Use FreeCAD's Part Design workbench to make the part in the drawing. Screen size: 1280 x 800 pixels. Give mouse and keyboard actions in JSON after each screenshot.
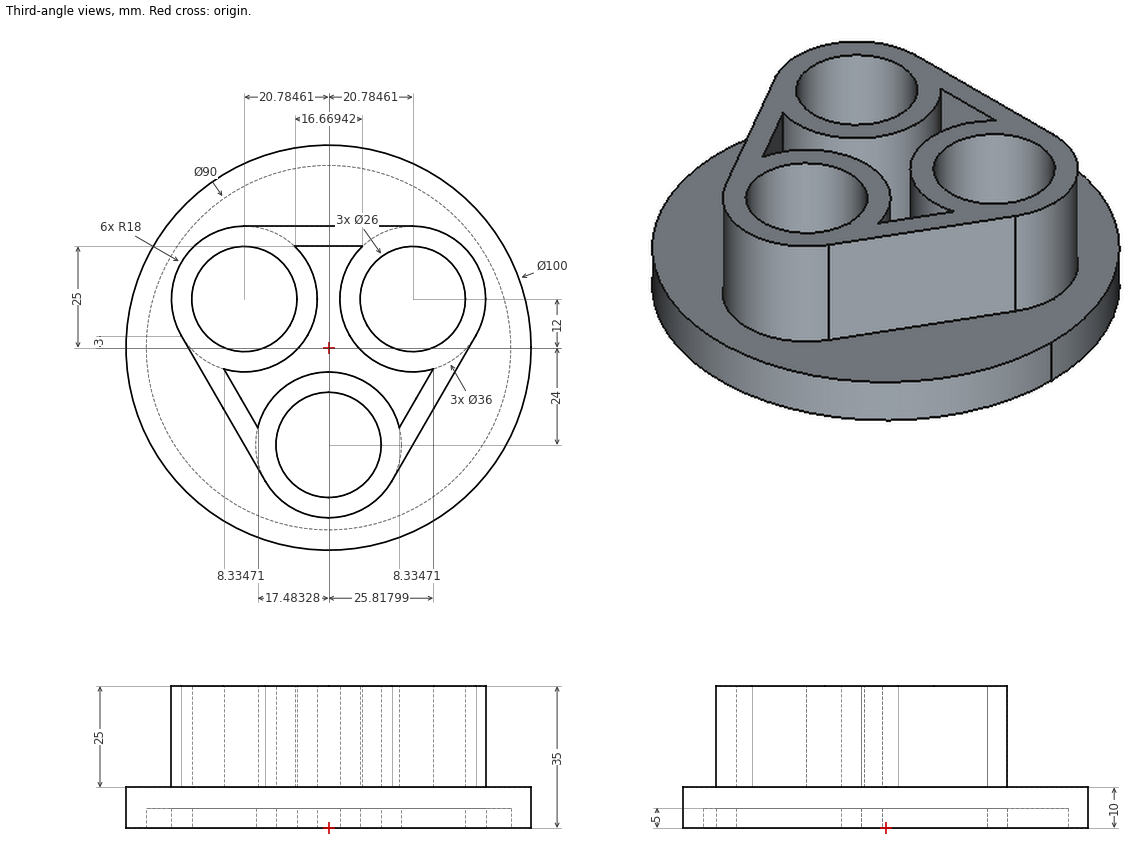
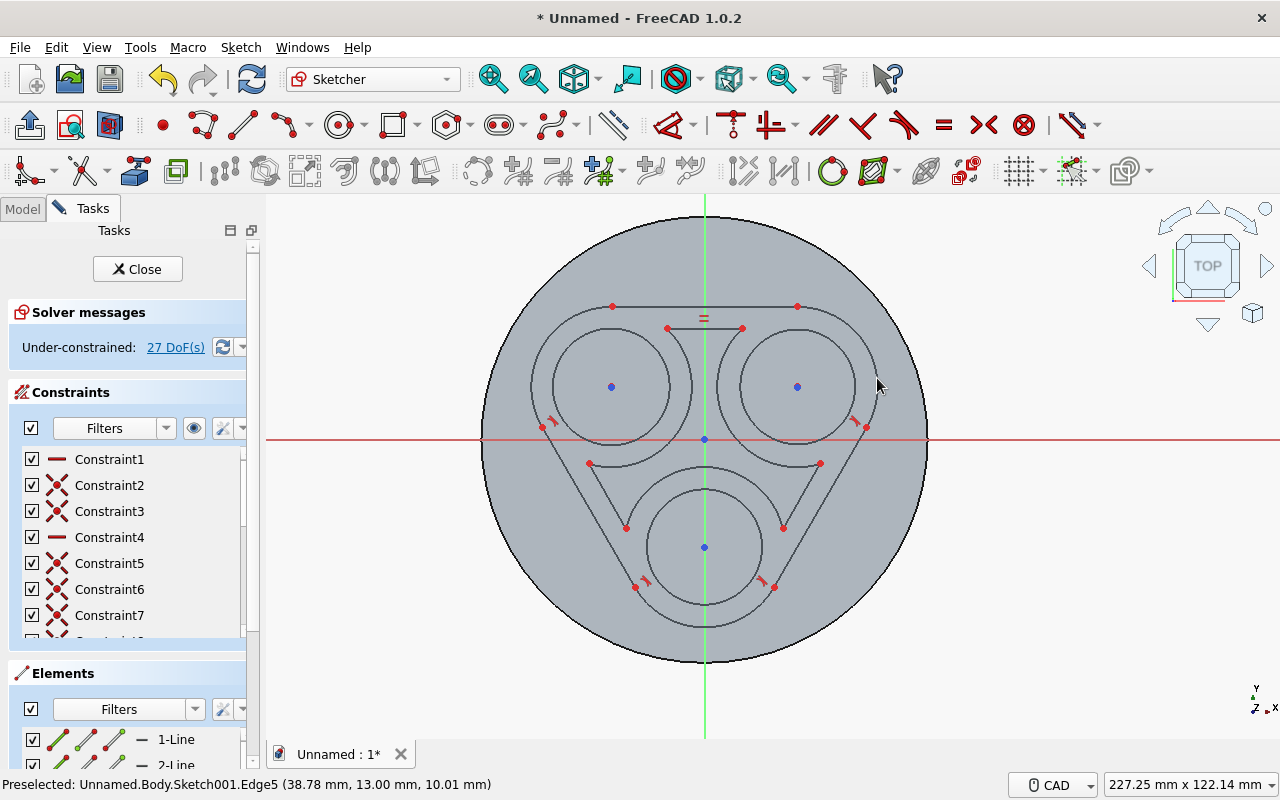
{"action": "left_click", "coordinate": [741, 307]}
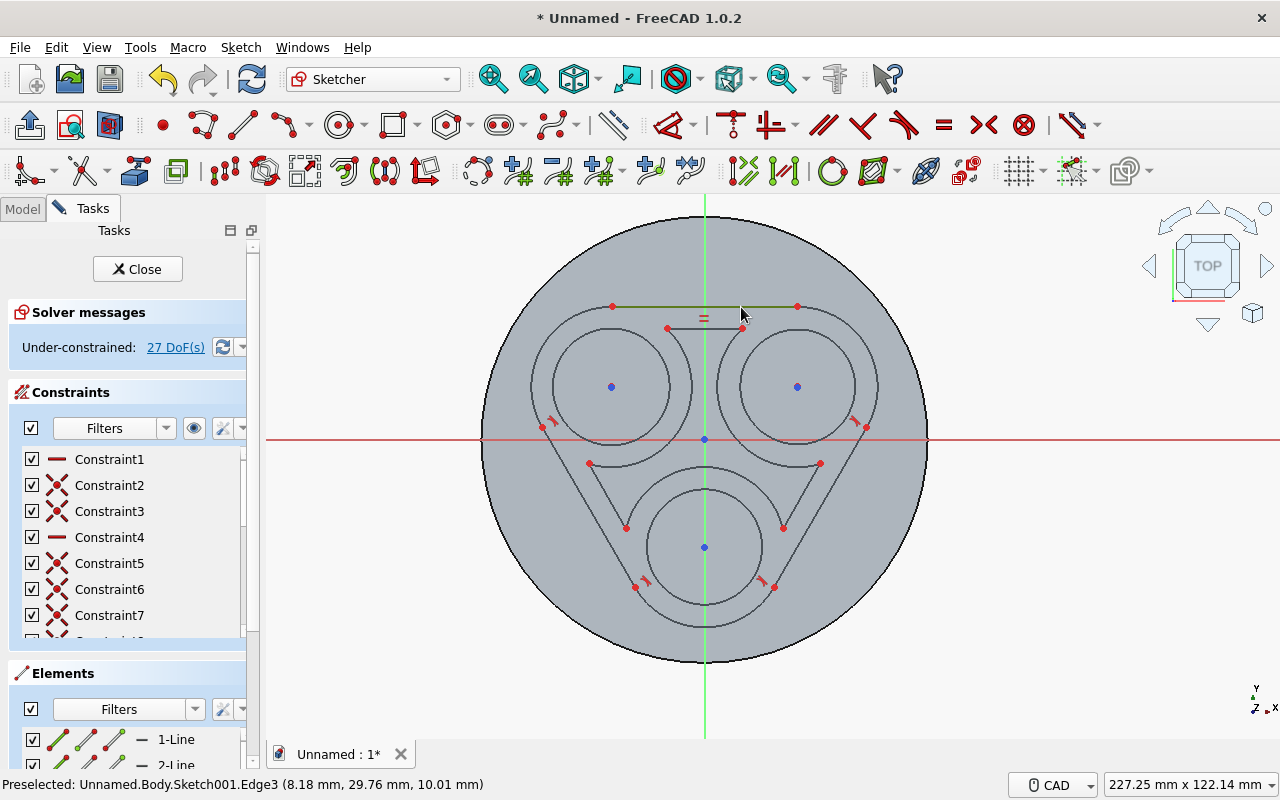
{"action": "left_click", "coordinate": [877, 378]}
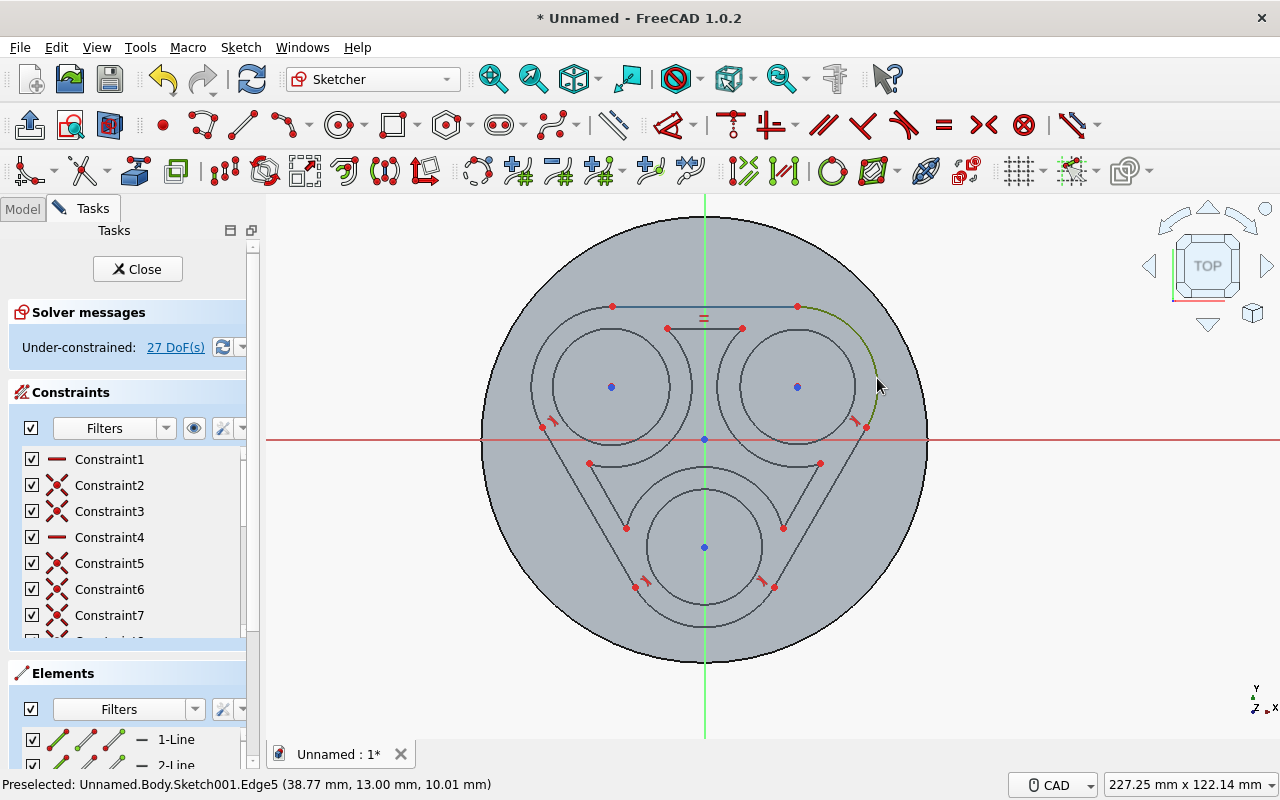
{"action": "left_click", "coordinate": [904, 126]}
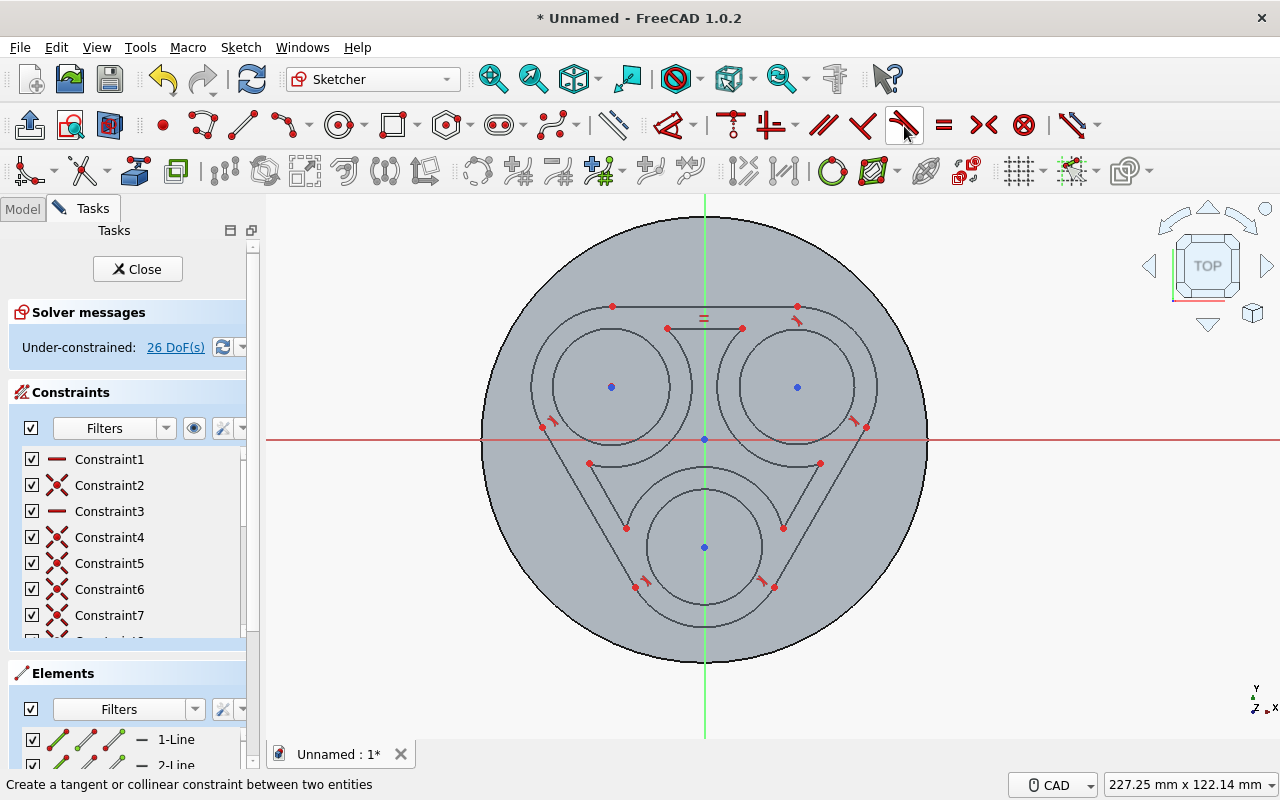
{"action": "left_click", "coordinate": [742, 307]}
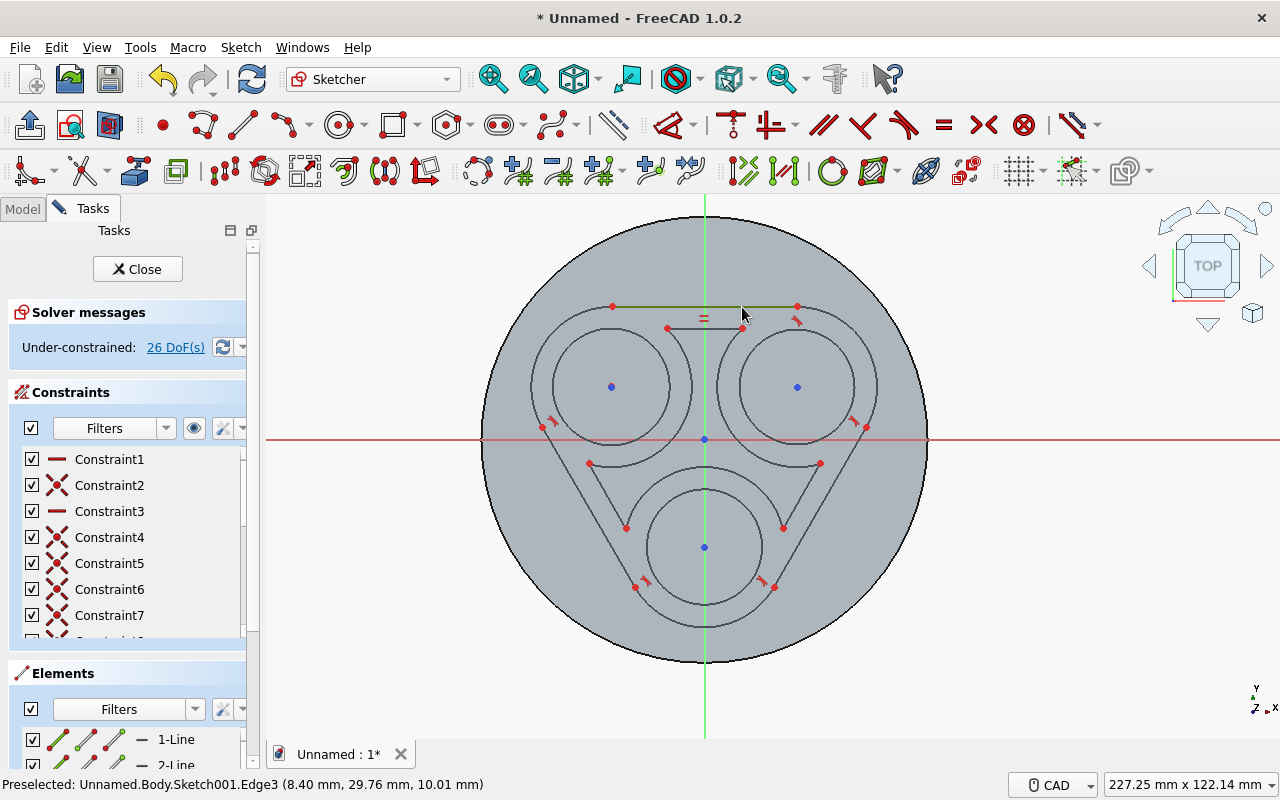
{"action": "left_click", "coordinate": [565, 322]}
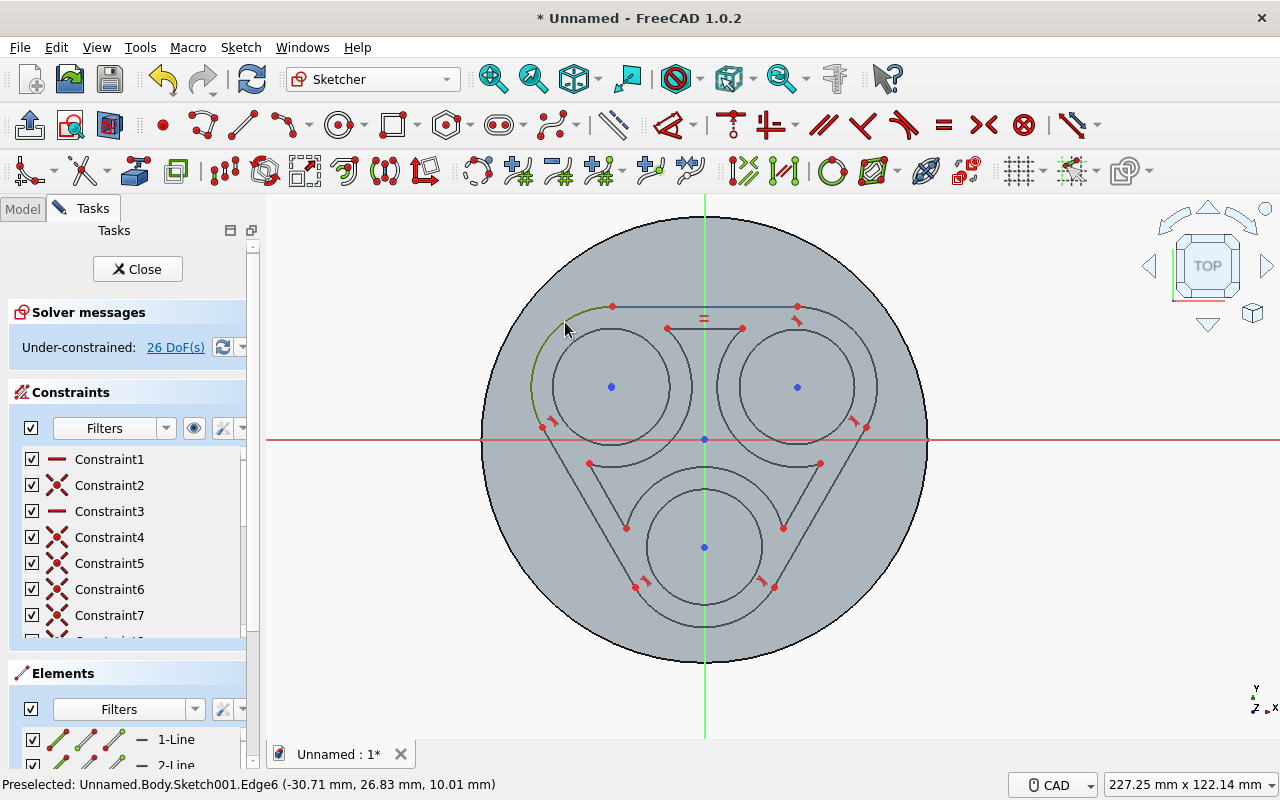
{"action": "left_click", "coordinate": [904, 126]}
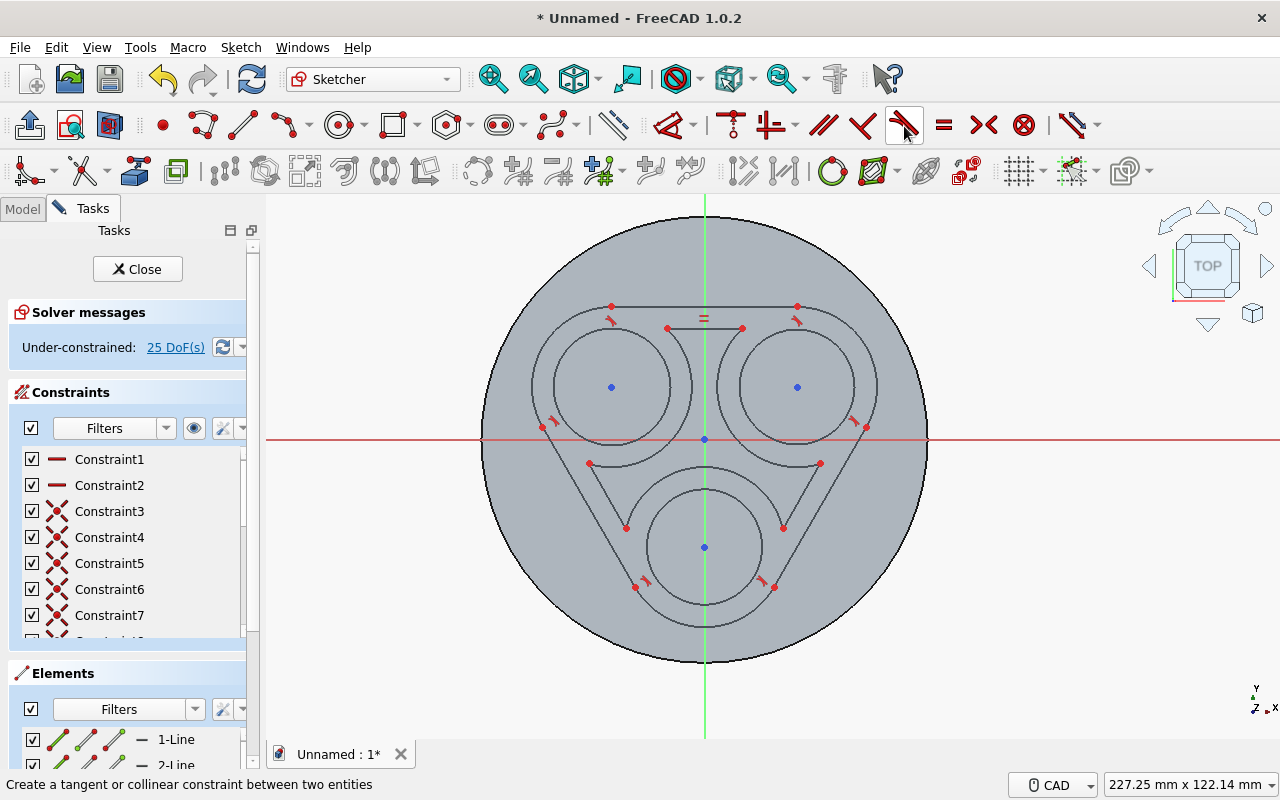
{"action": "left_click", "coordinate": [653, 346]}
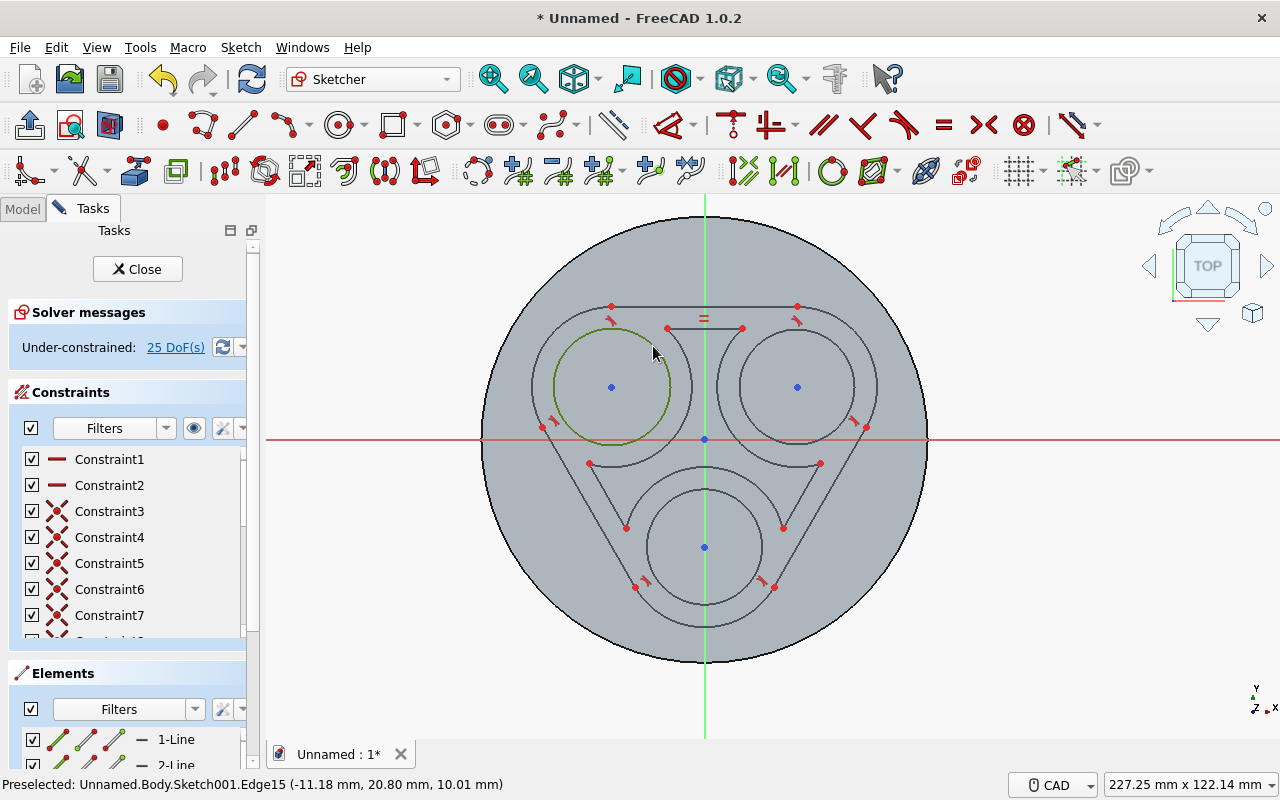
{"action": "left_click", "coordinate": [651, 457]}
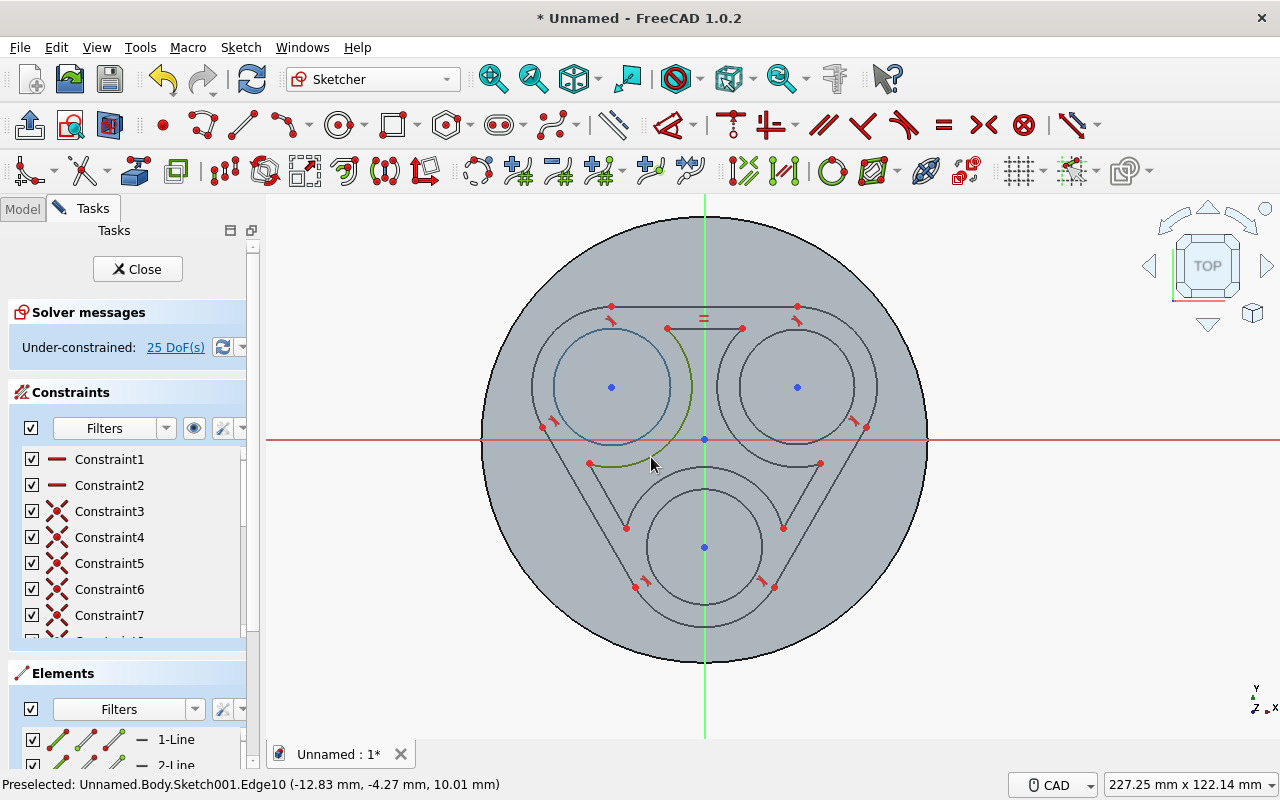
{"action": "key", "text": "c"}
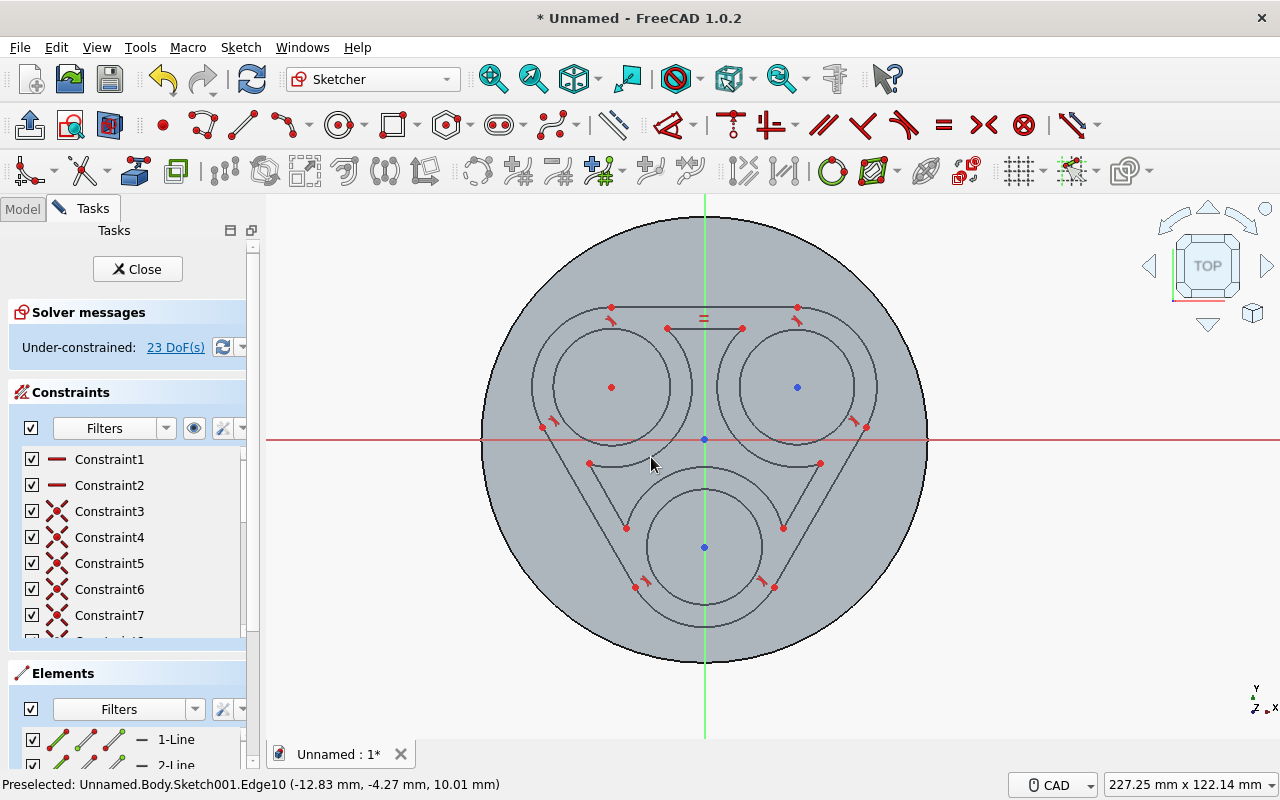
{"action": "left_click", "coordinate": [838, 346]}